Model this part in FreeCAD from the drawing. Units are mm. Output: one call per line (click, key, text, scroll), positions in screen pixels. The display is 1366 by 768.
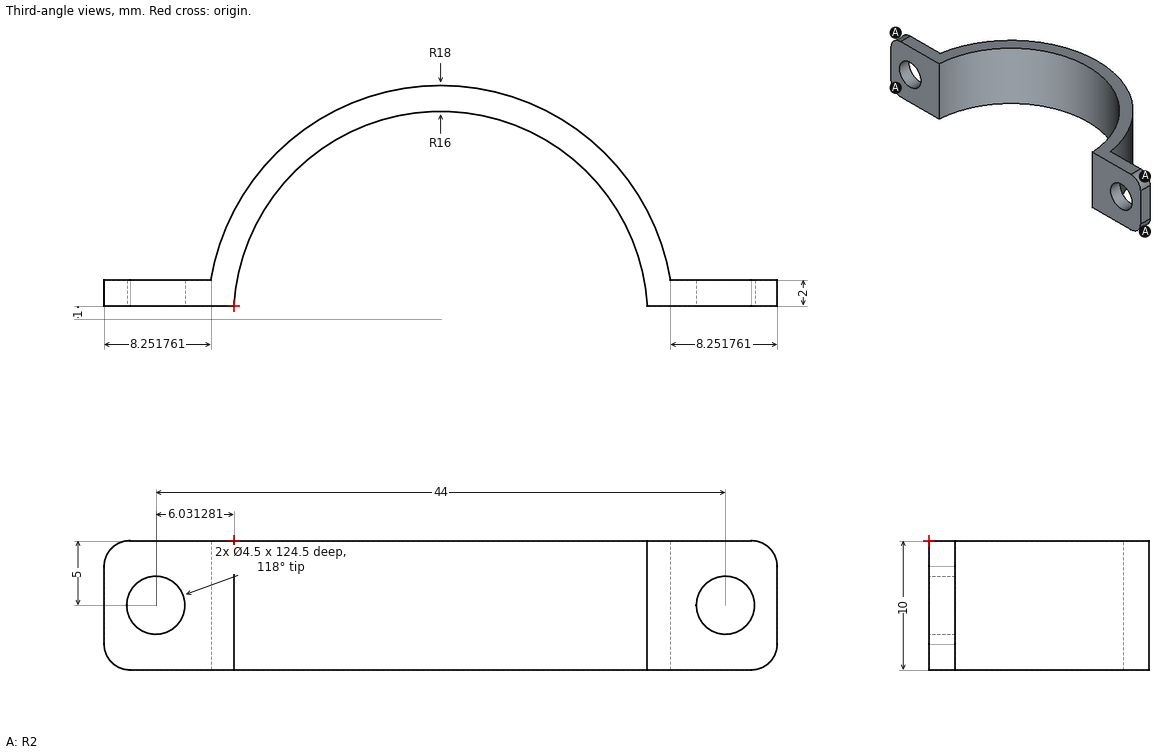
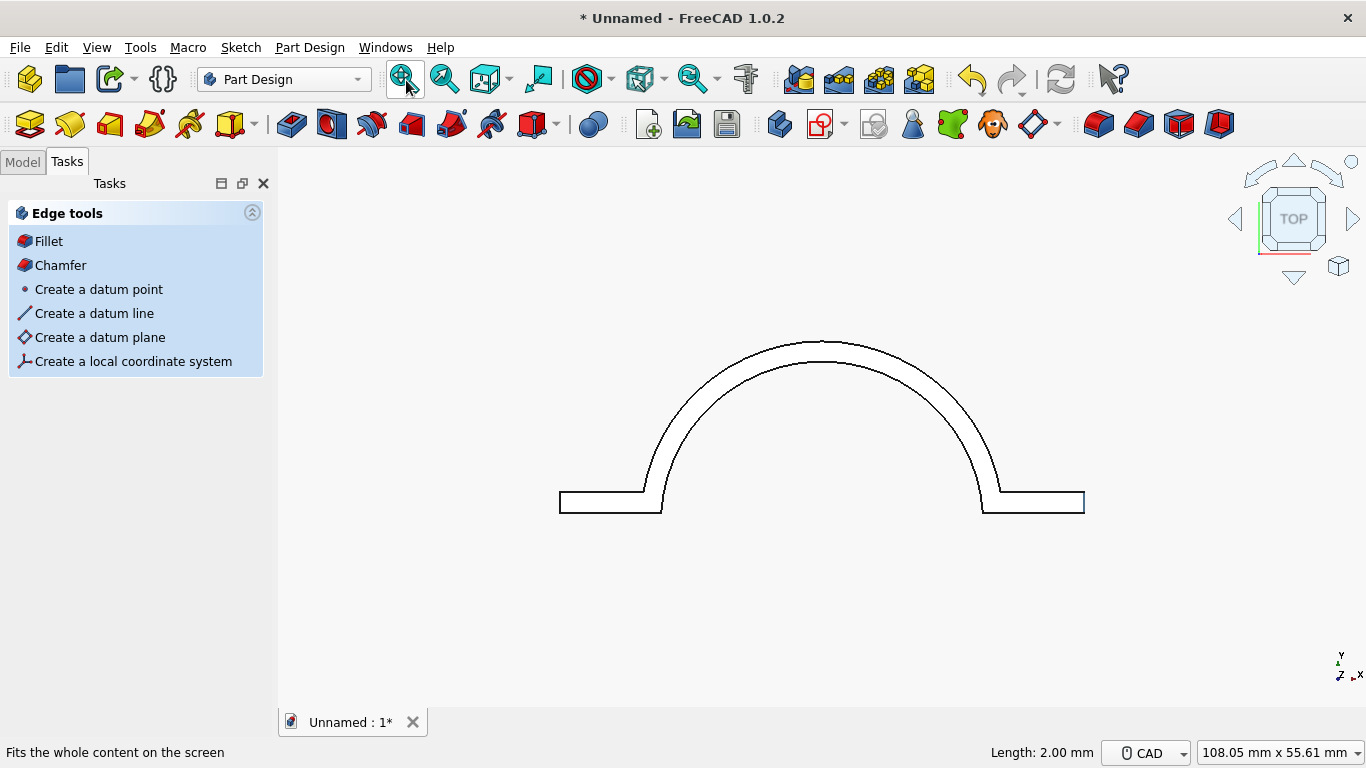
click(560, 502, ctrl)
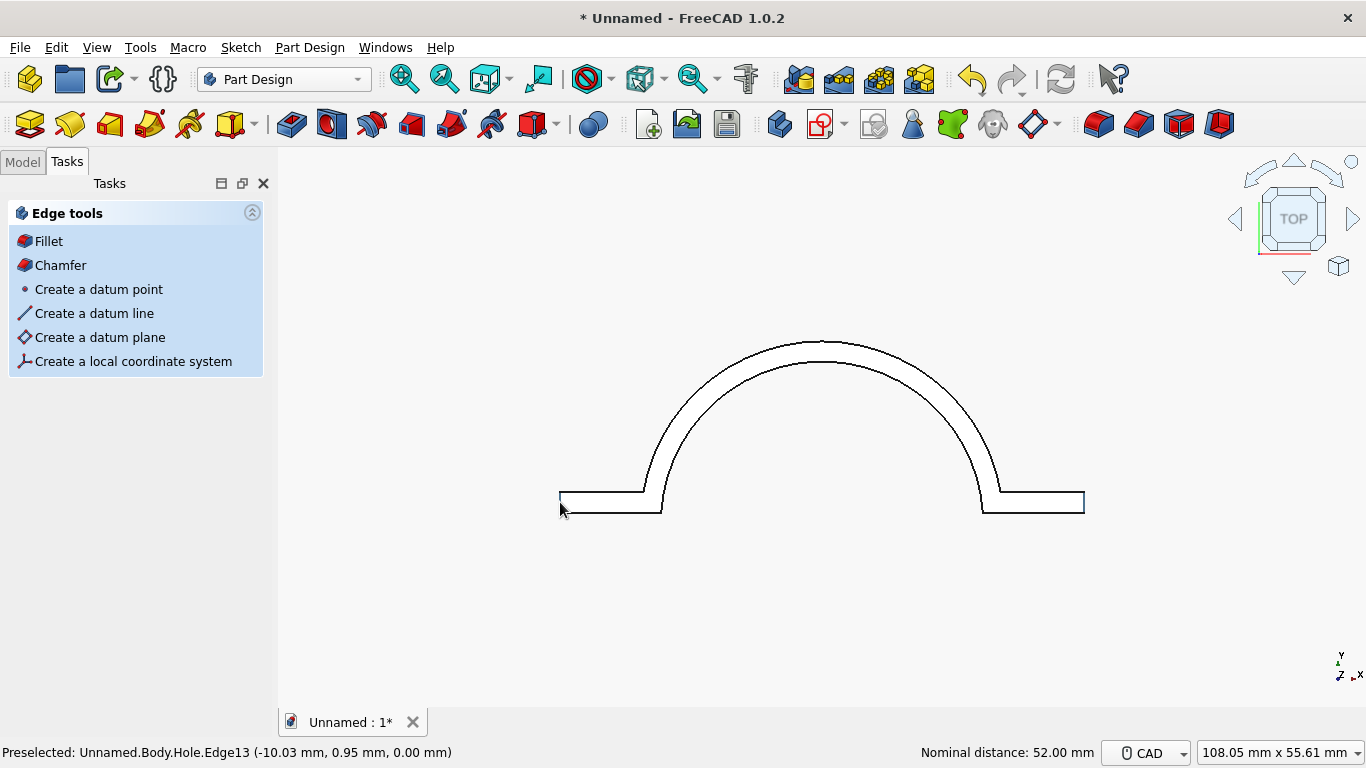
scroll(560, 502, up, 4)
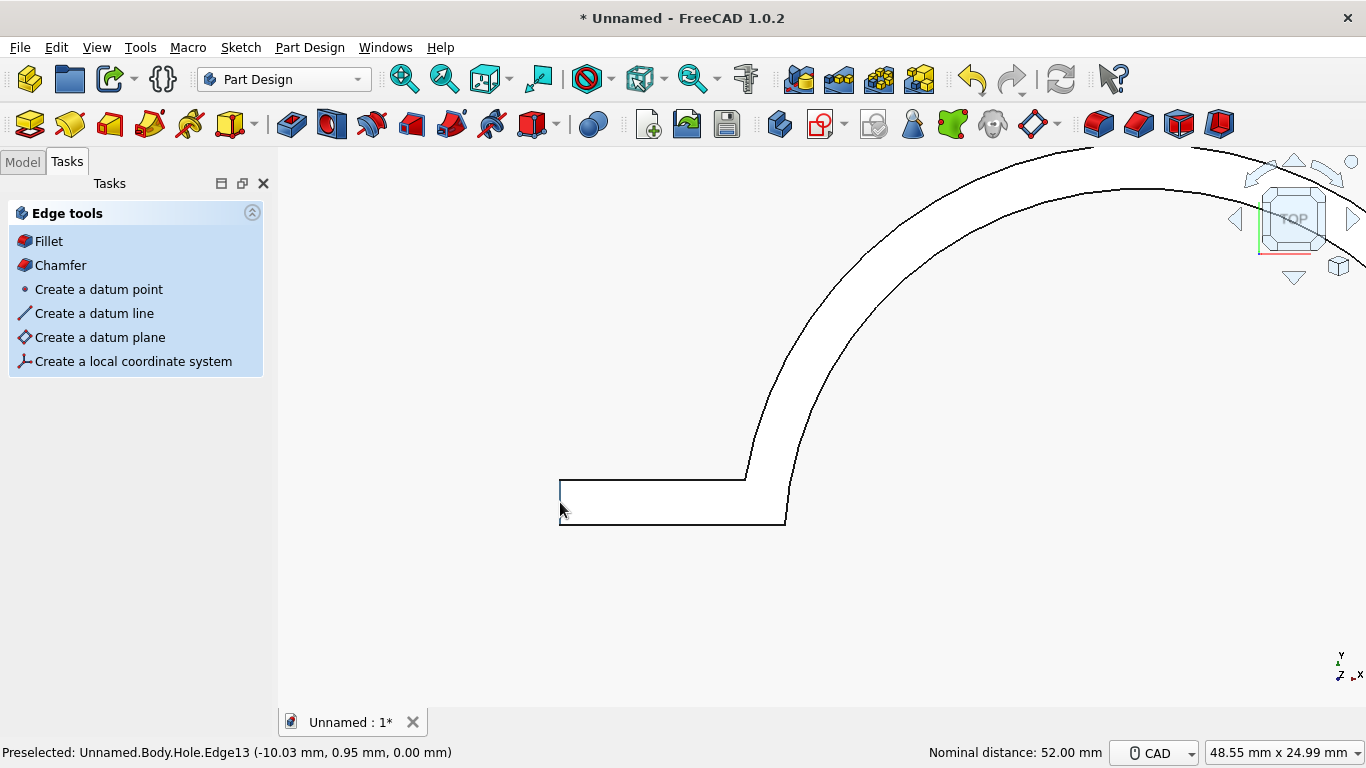
click(406, 80)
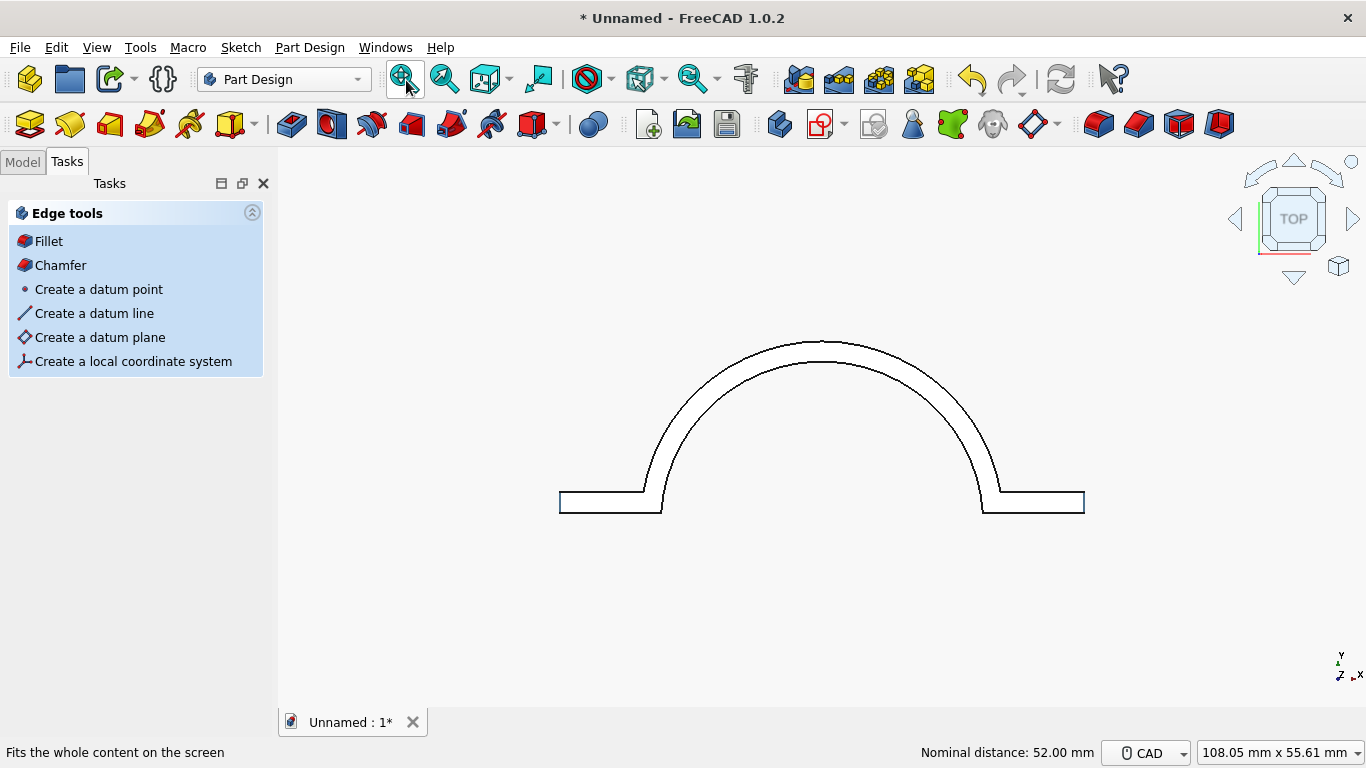
key(1)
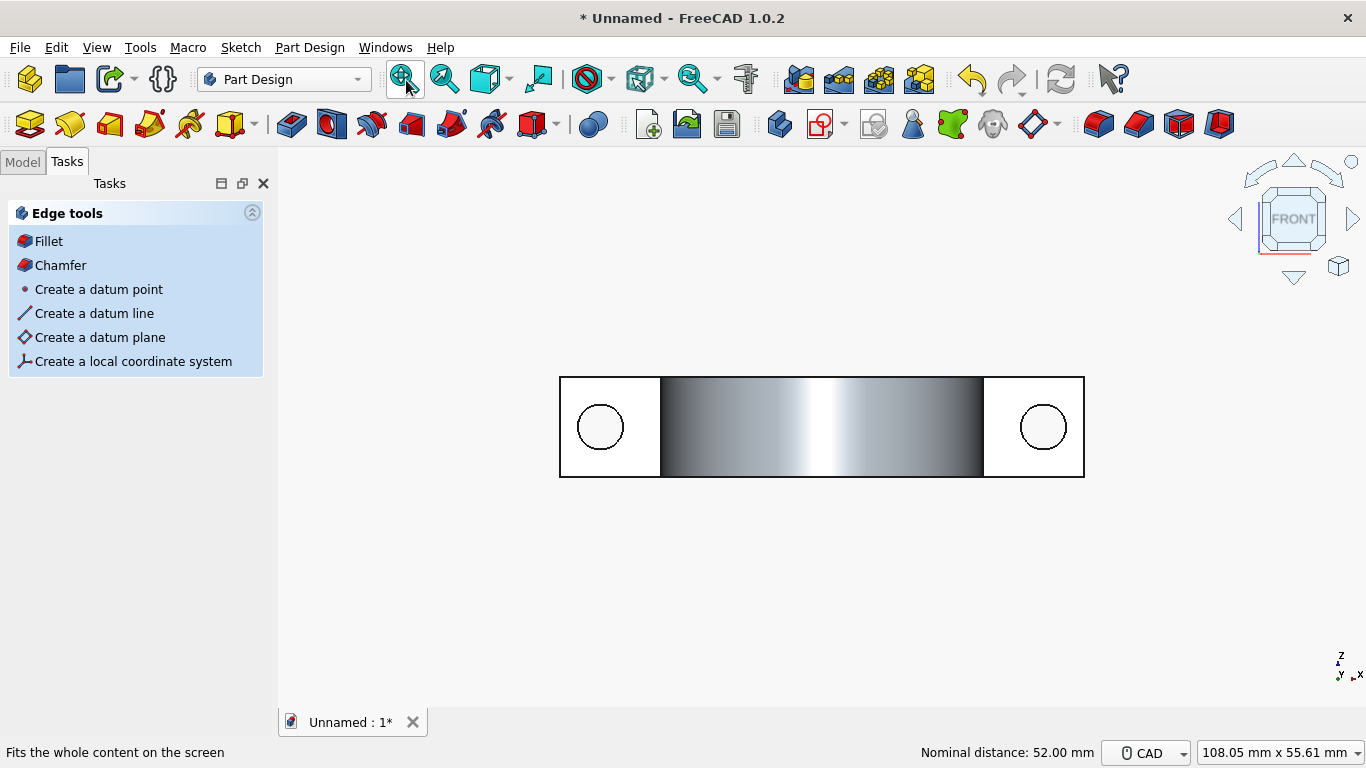
scroll(560, 476, up, 4)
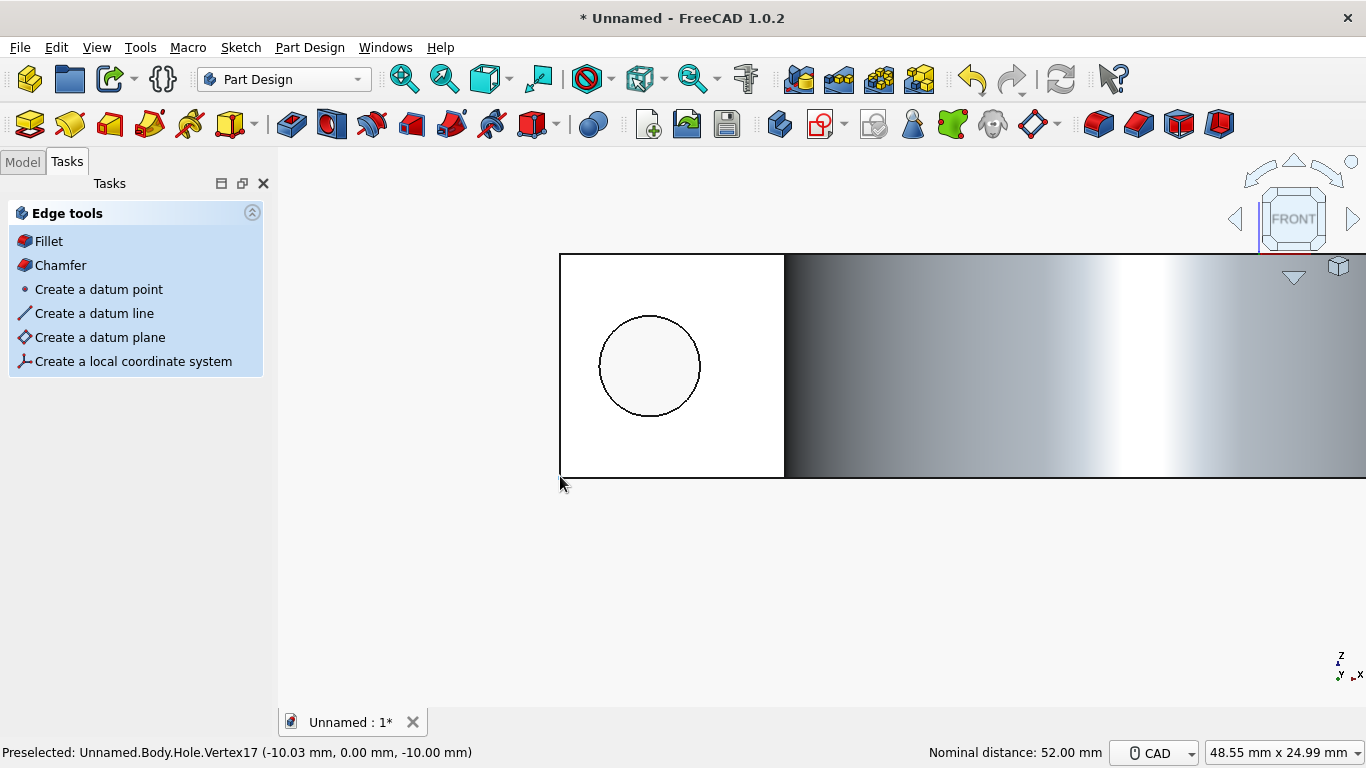
click(406, 80)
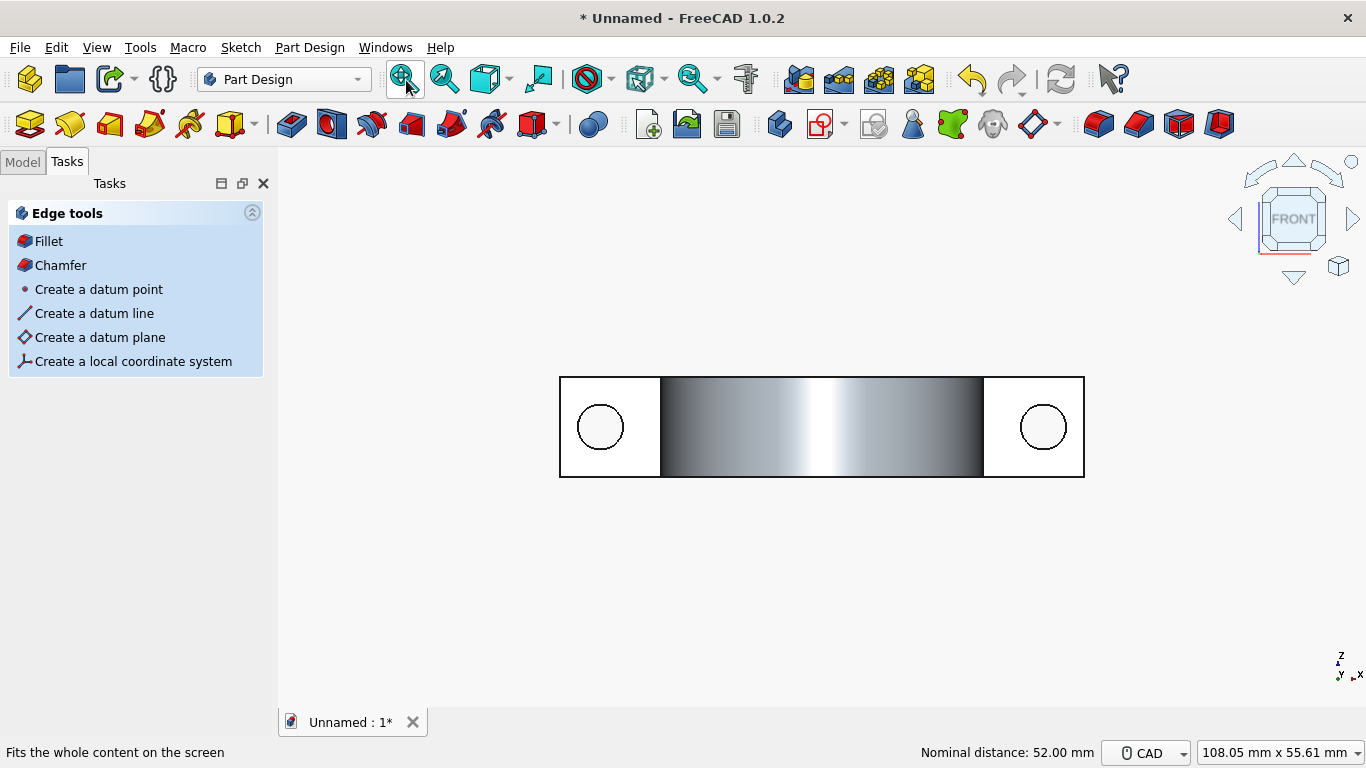
key(3)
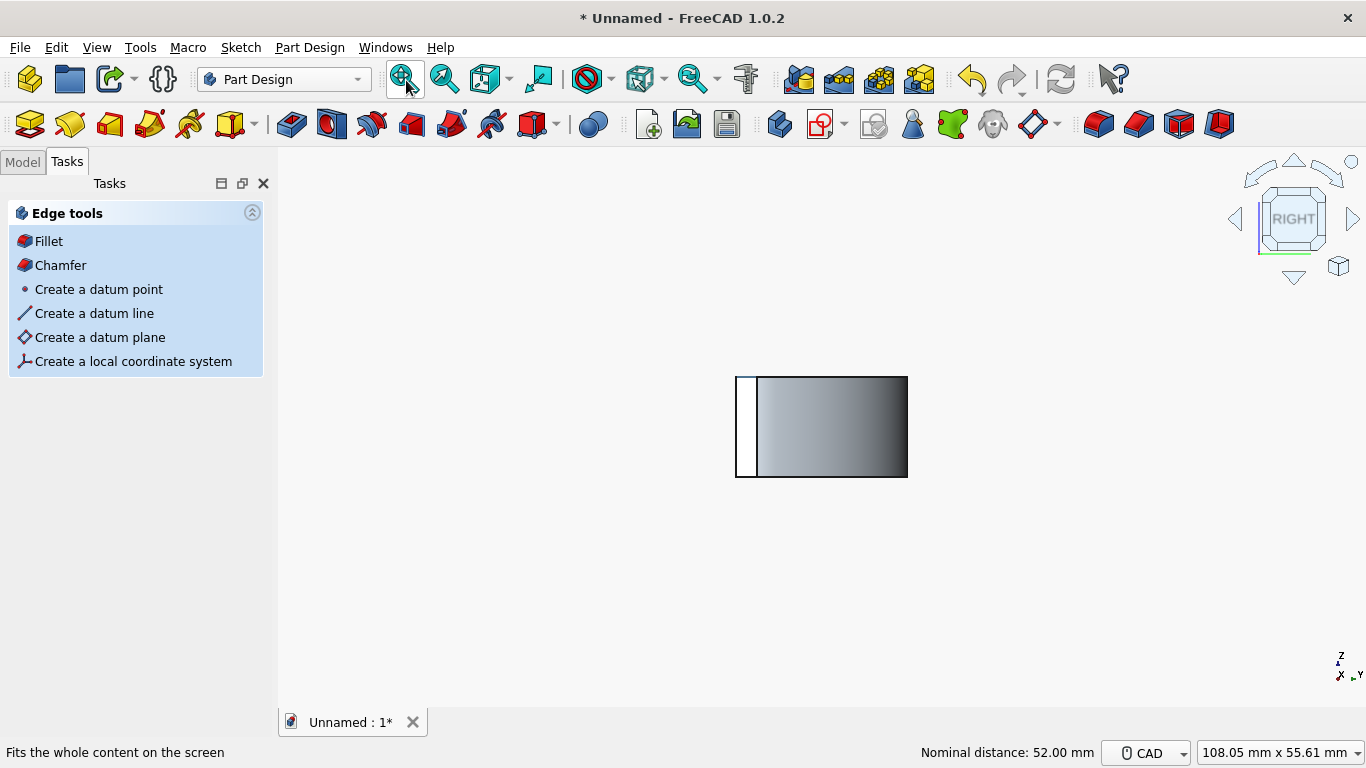
click(406, 80)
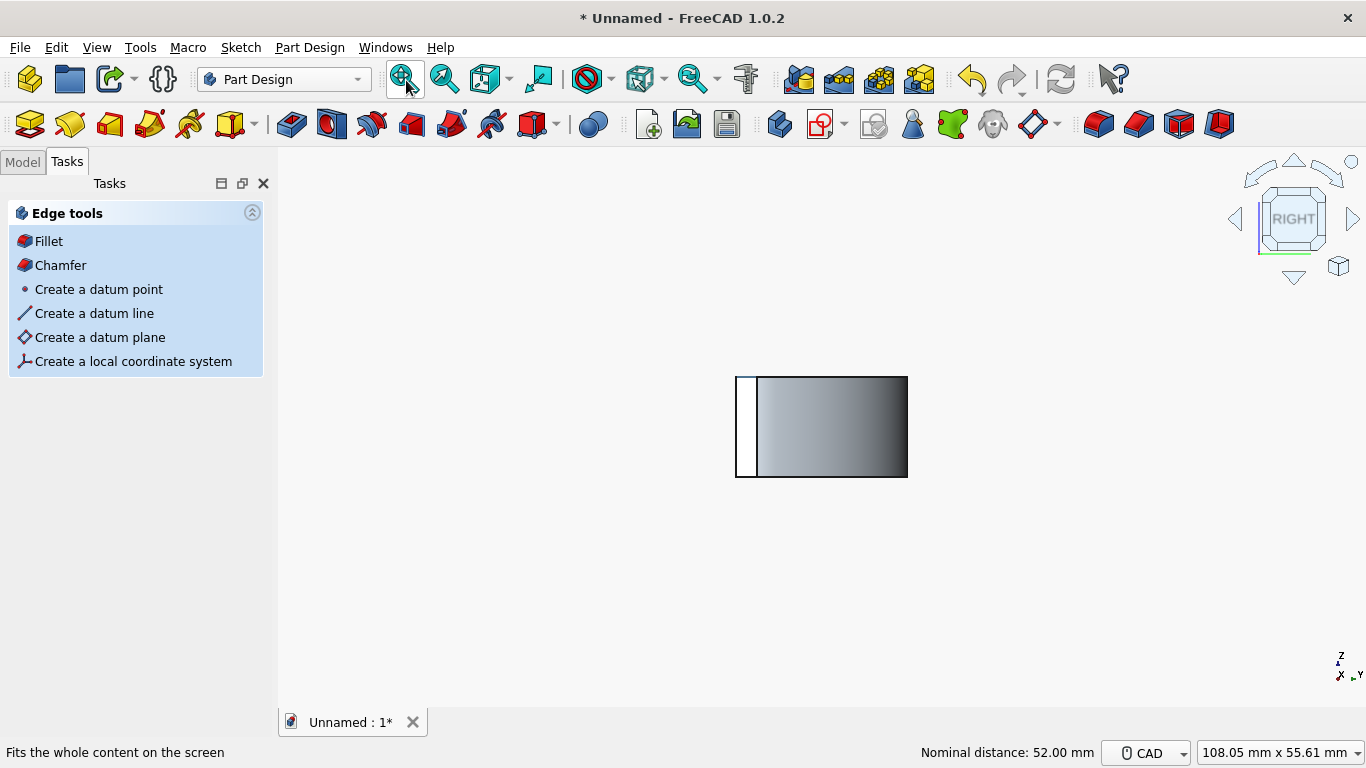
click(746, 476, ctrl)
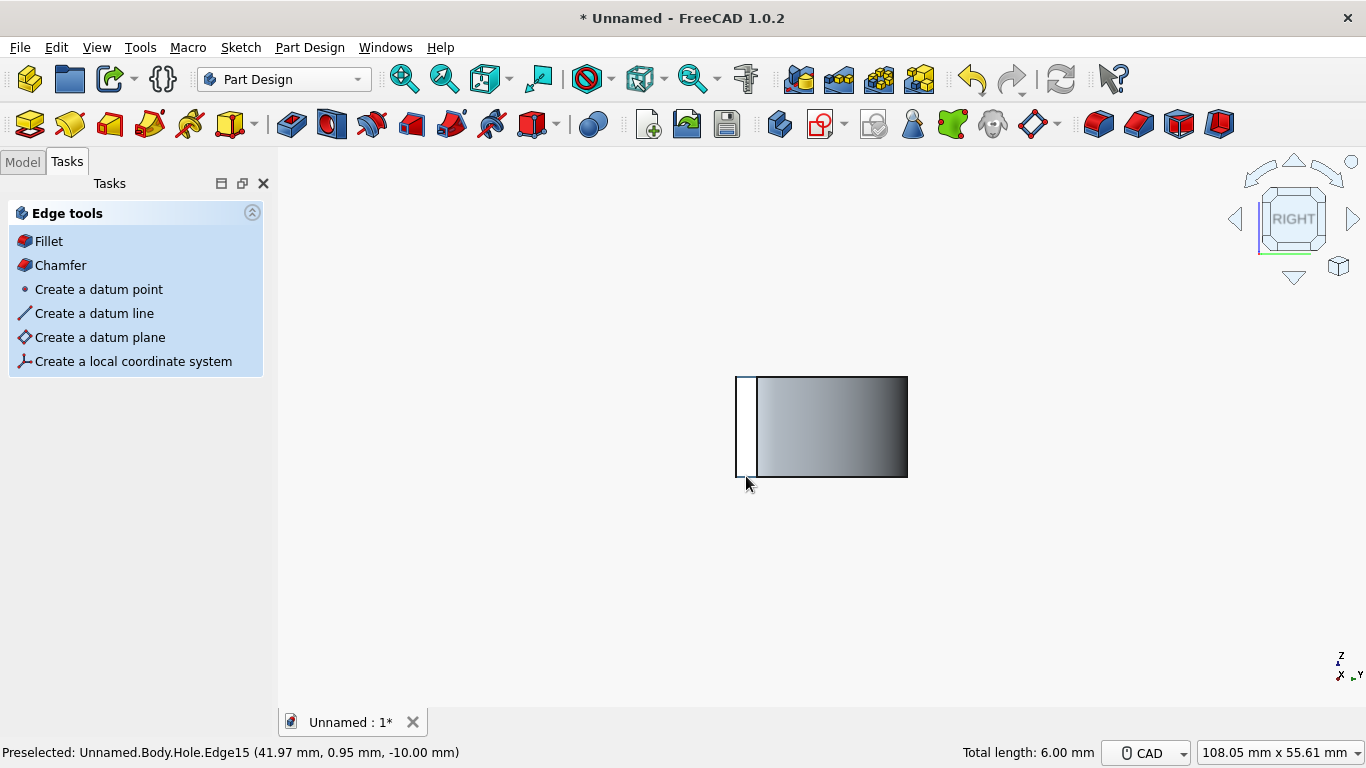
scroll(746, 476, up, 4)